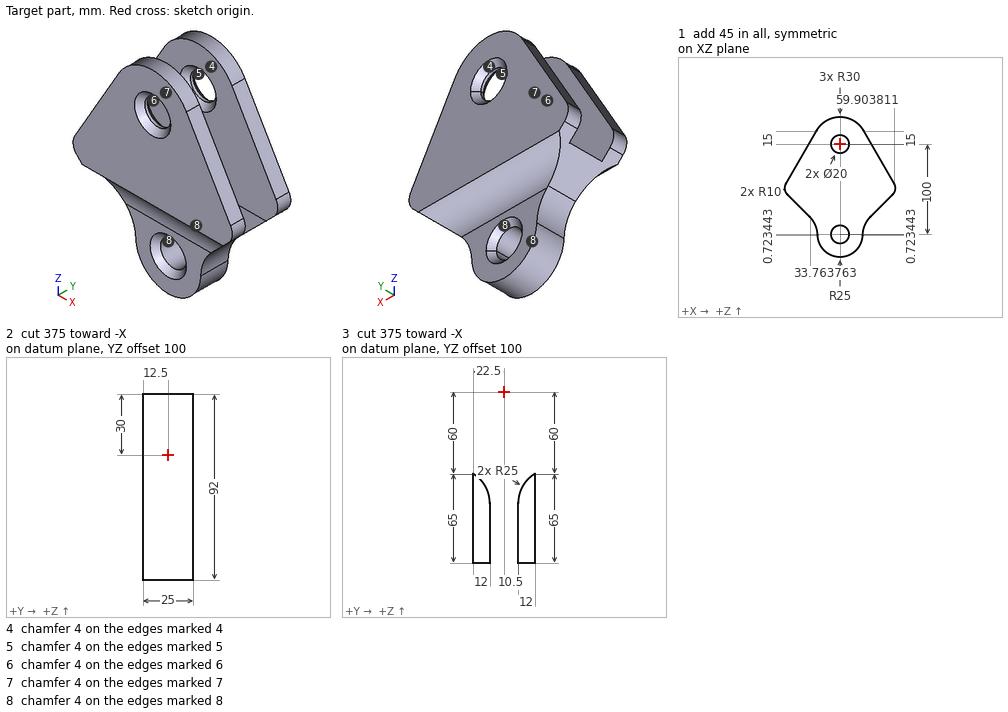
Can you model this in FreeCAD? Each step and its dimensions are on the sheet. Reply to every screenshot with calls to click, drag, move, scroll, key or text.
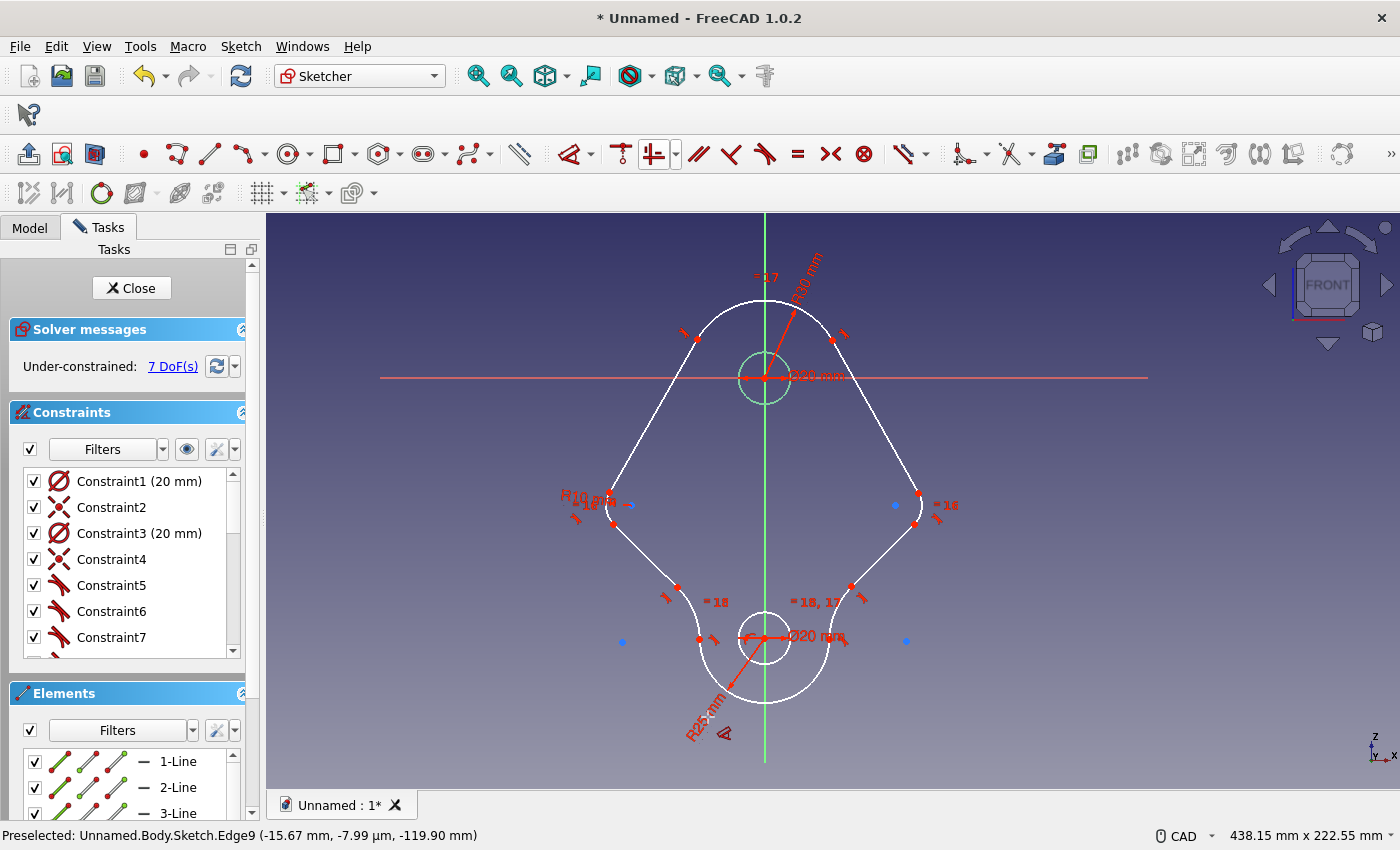
click(697, 340)
click(663, 359)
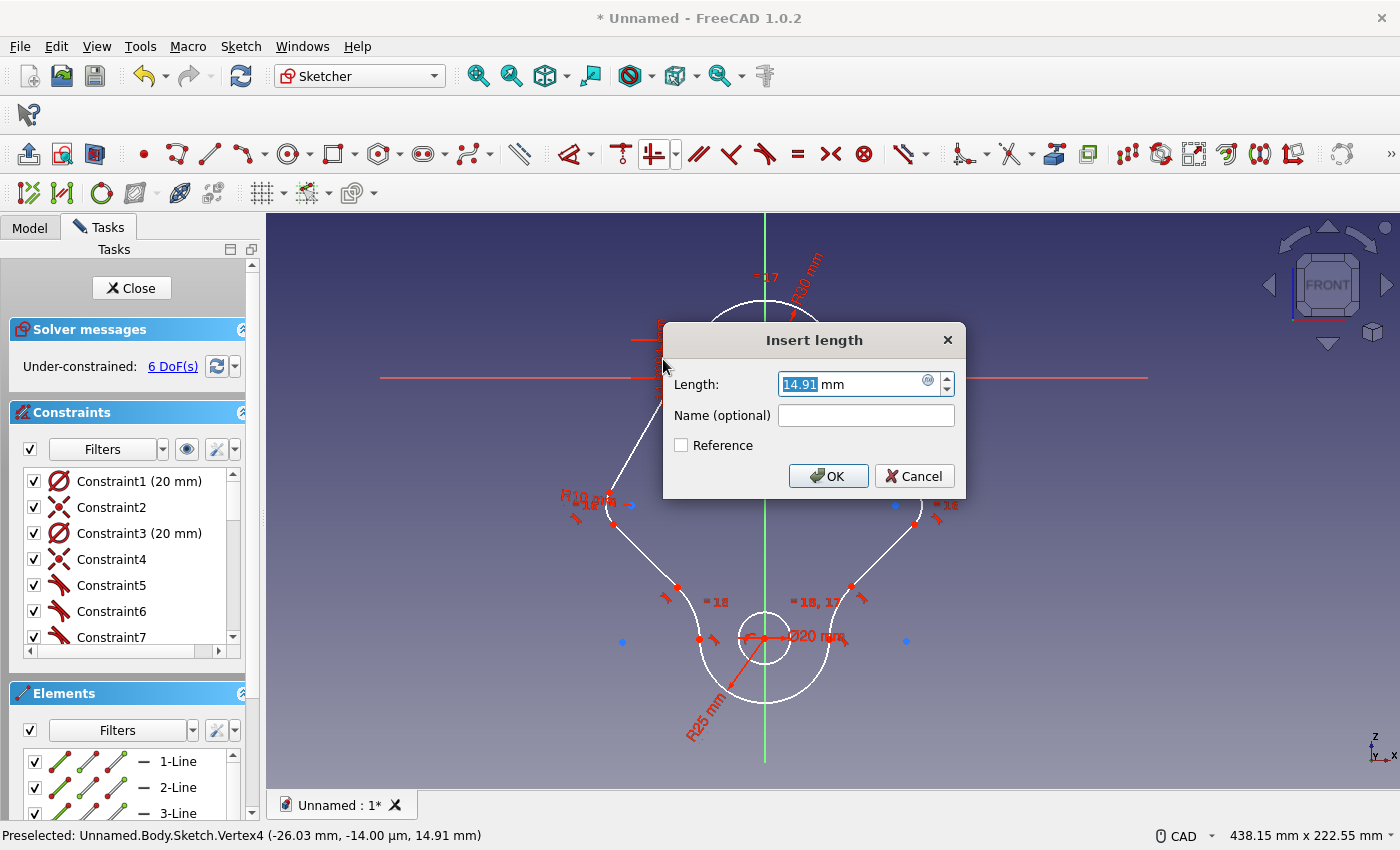
text(15)
key(Return)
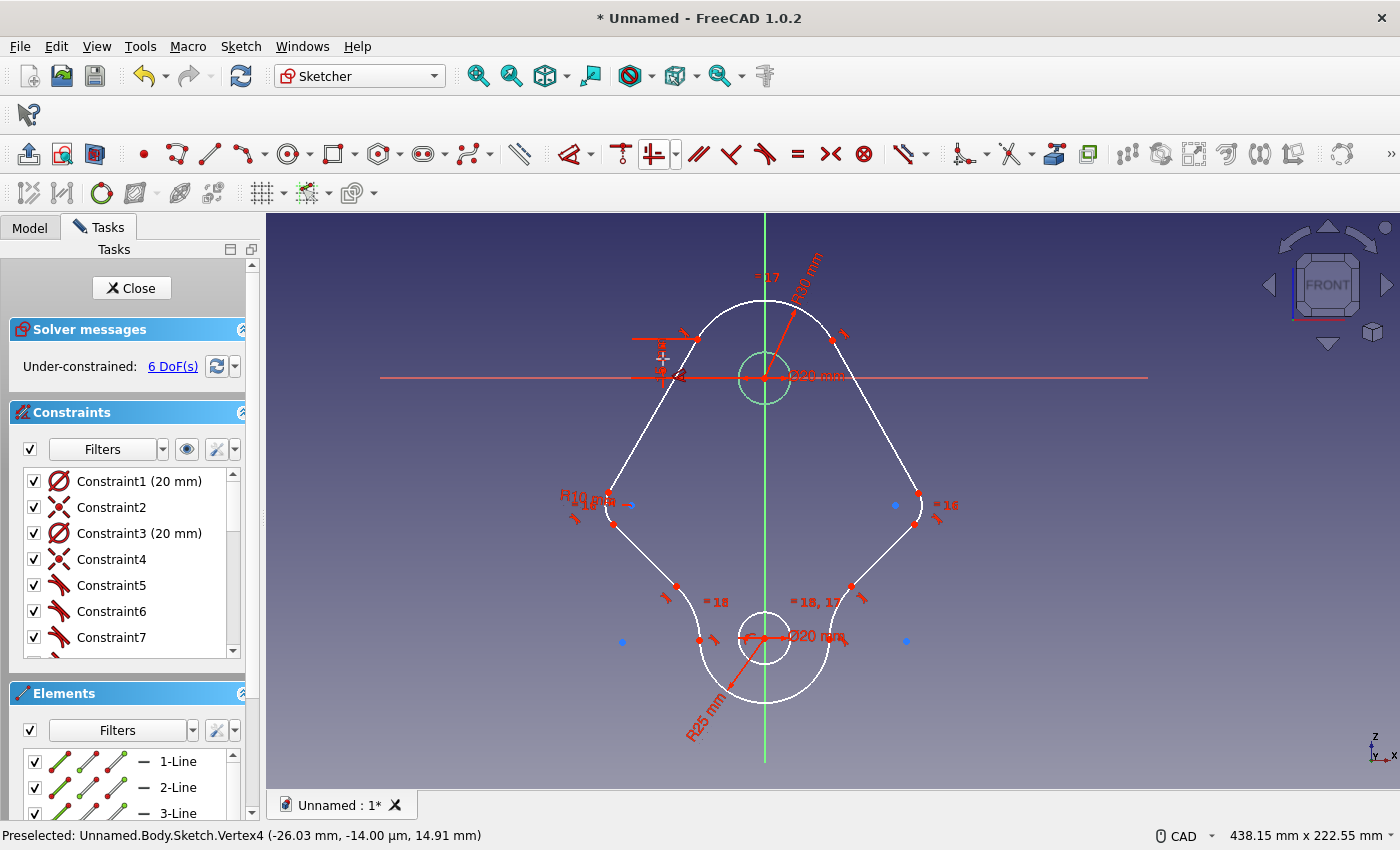
click(832, 340)
click(866, 359)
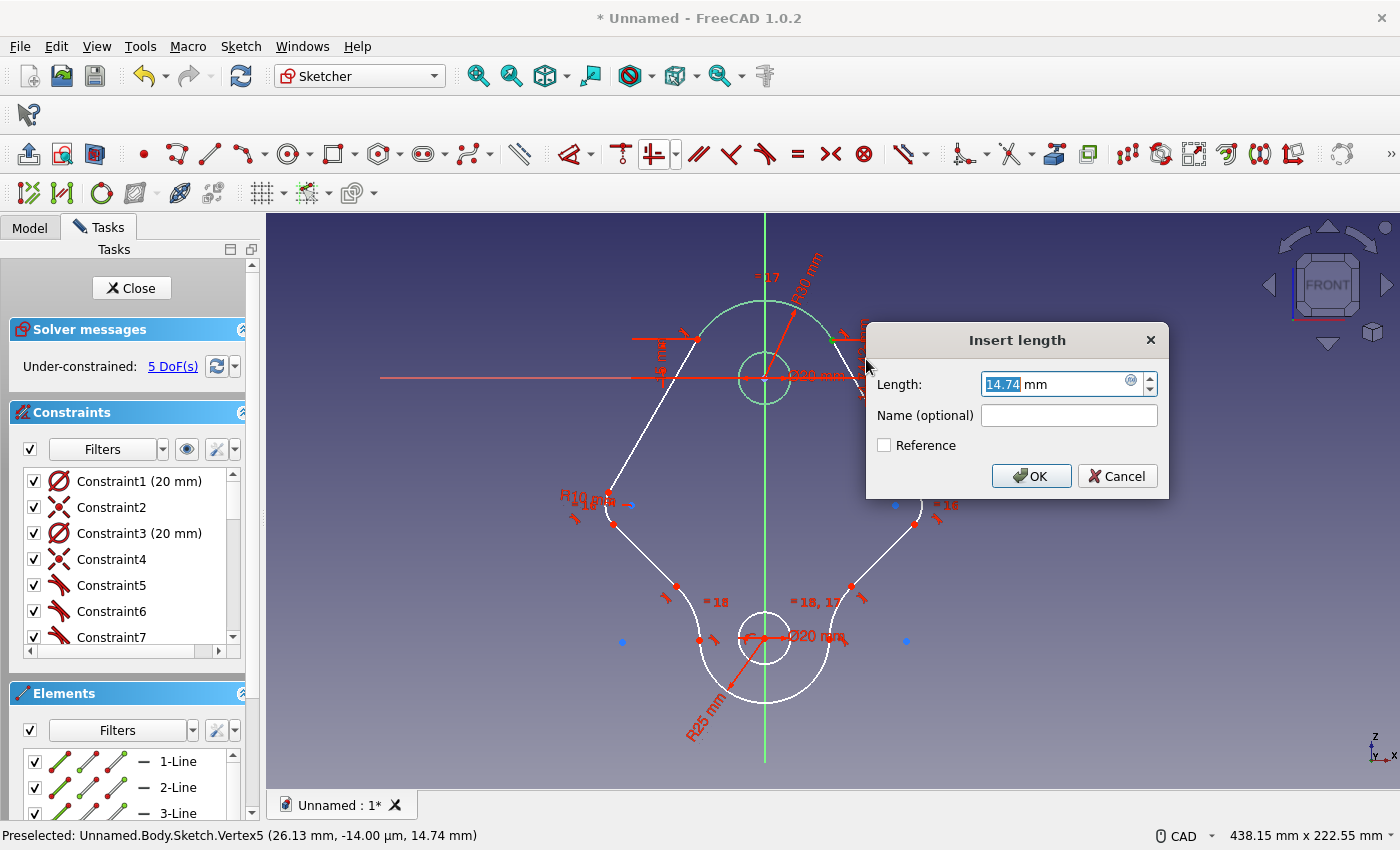
text(15)
key(Return)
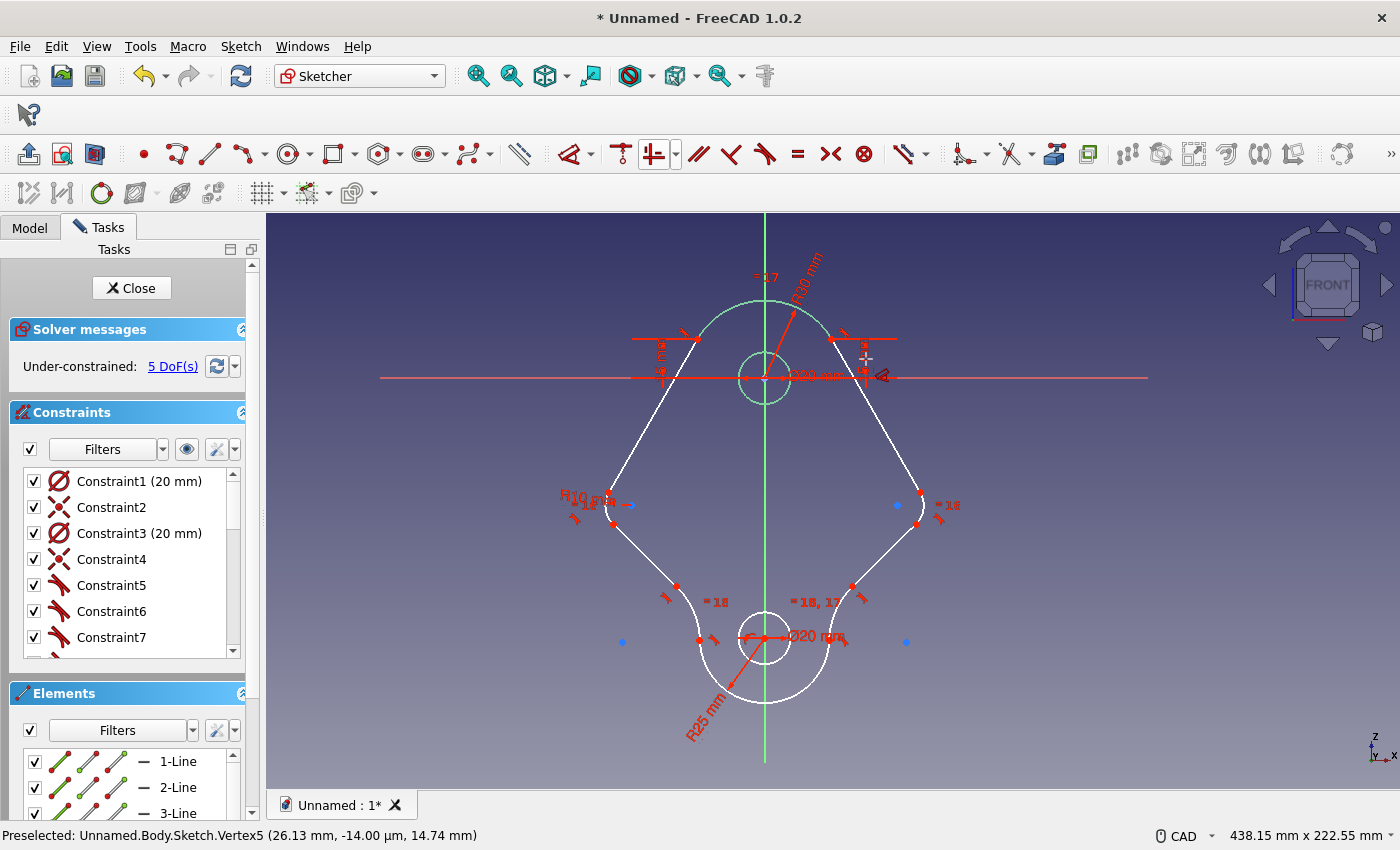
click(765, 638)
click(799, 508)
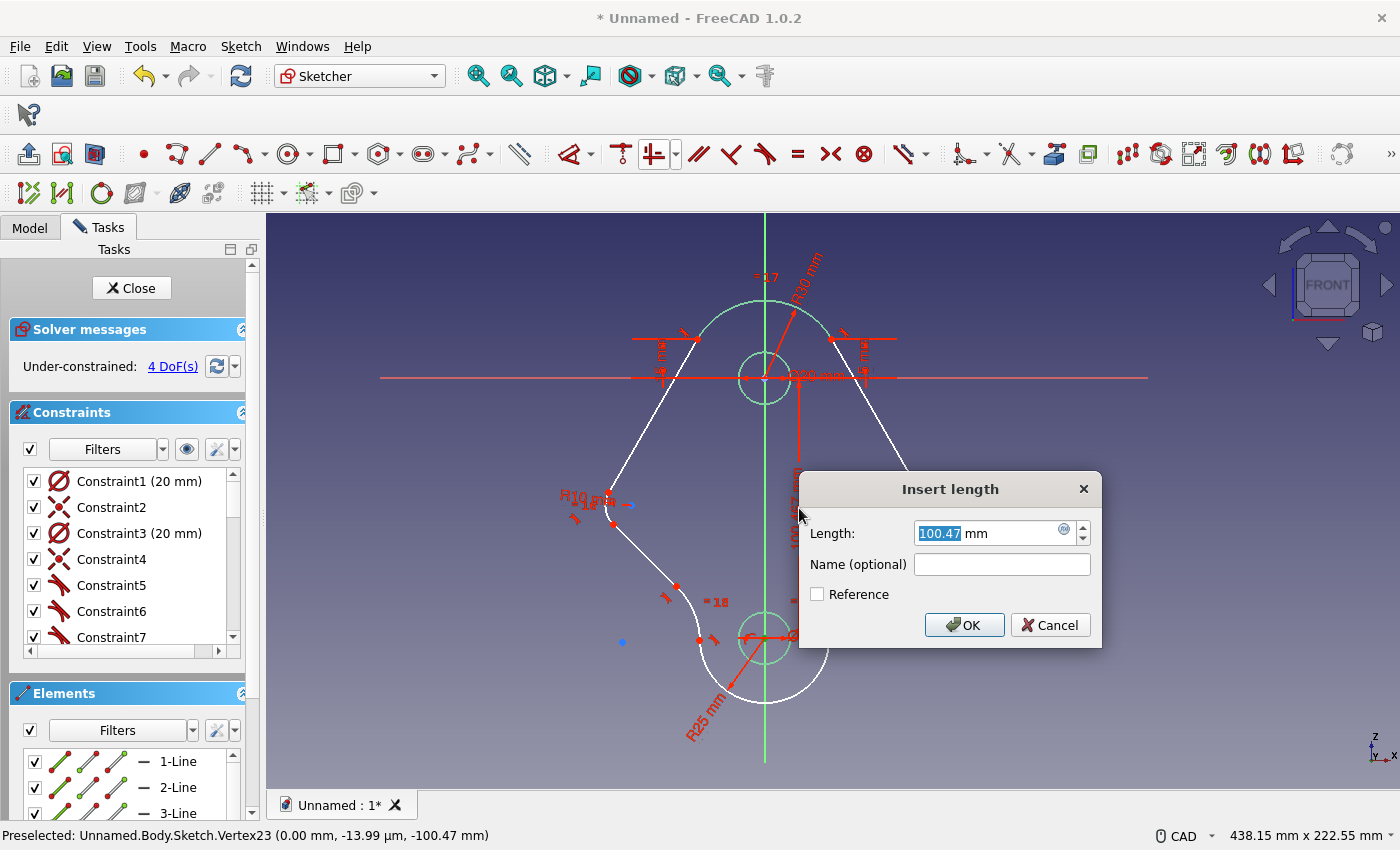
text(100)
key(Return)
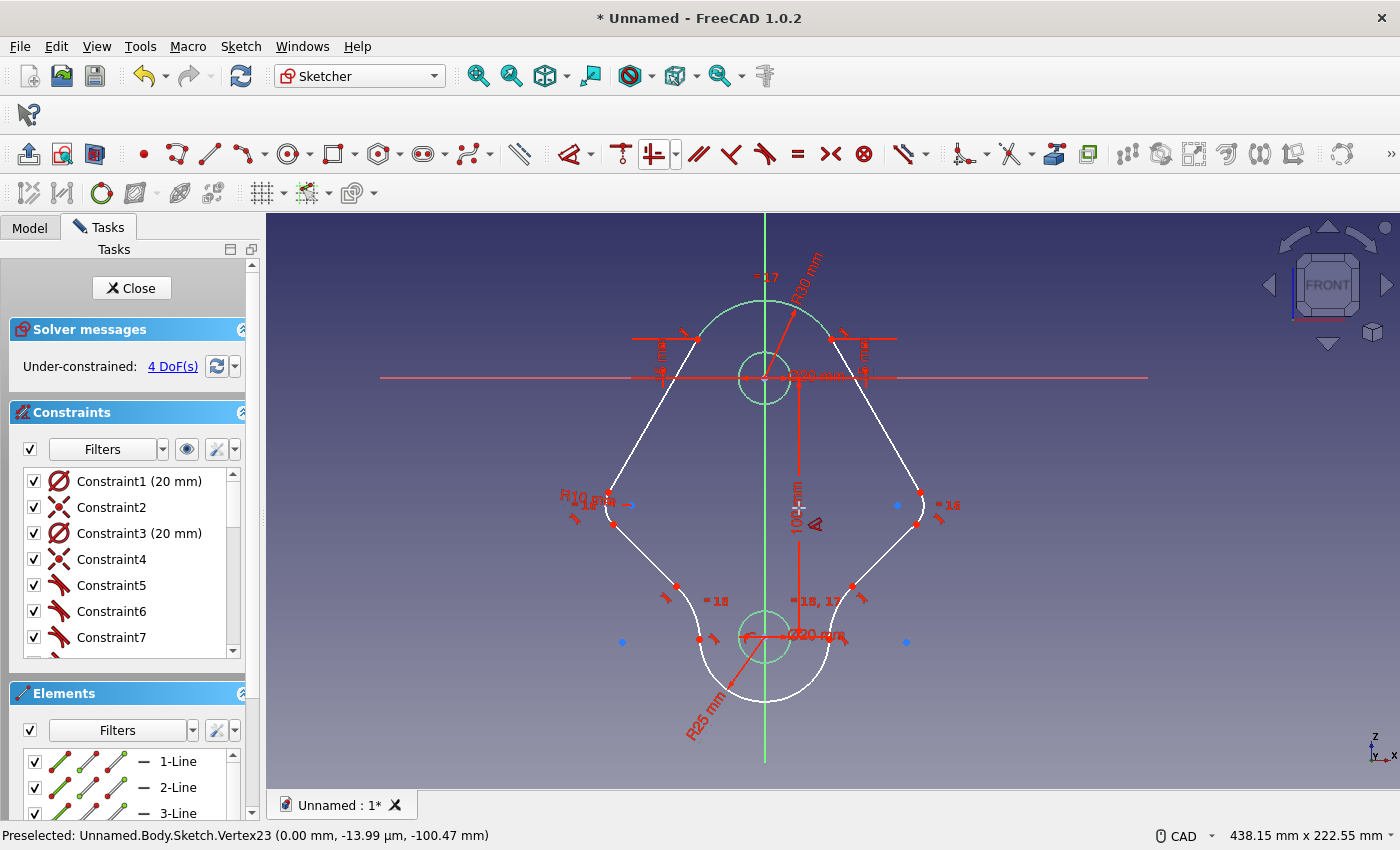
scroll(829, 639, up, 16)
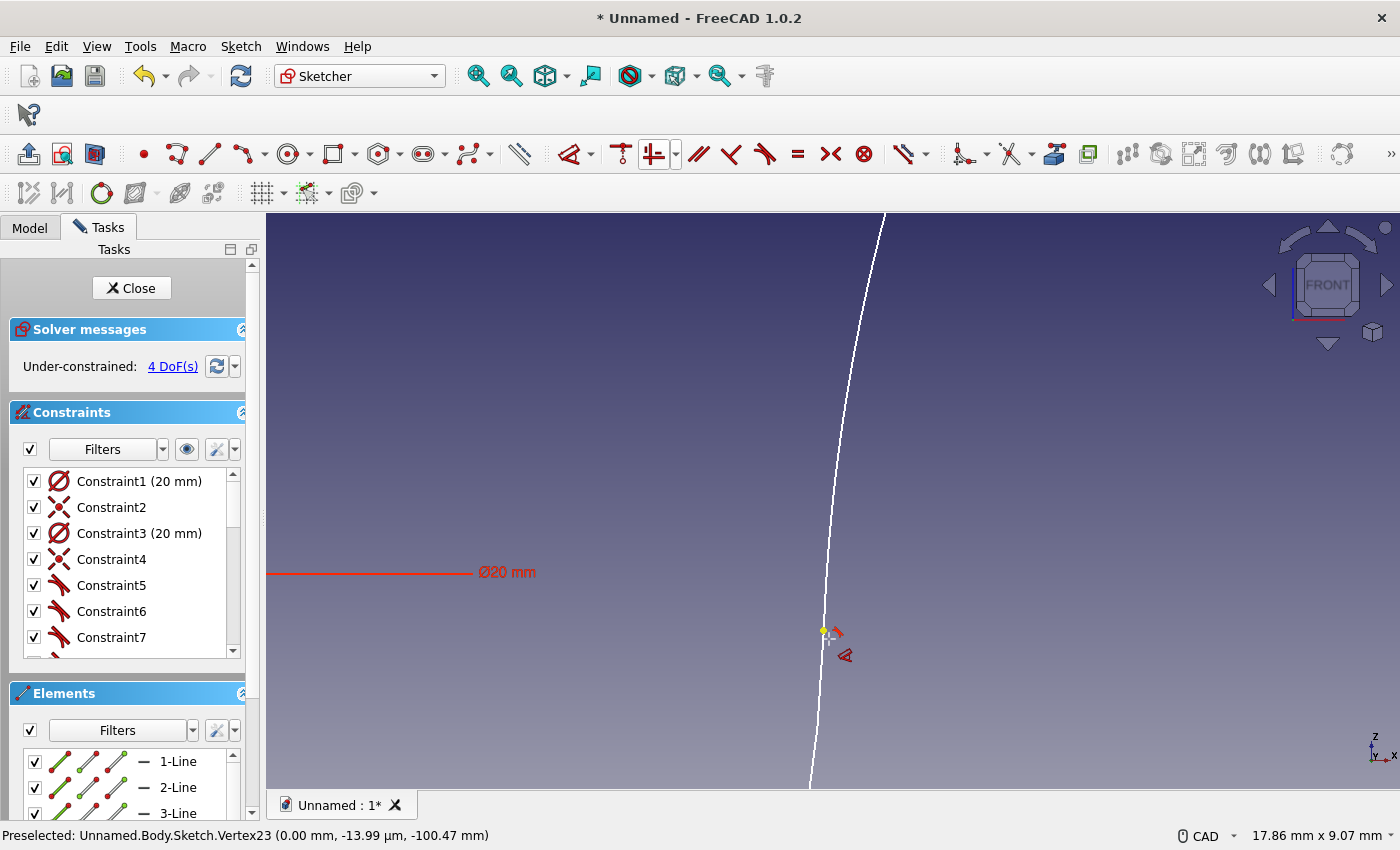
click(824, 631)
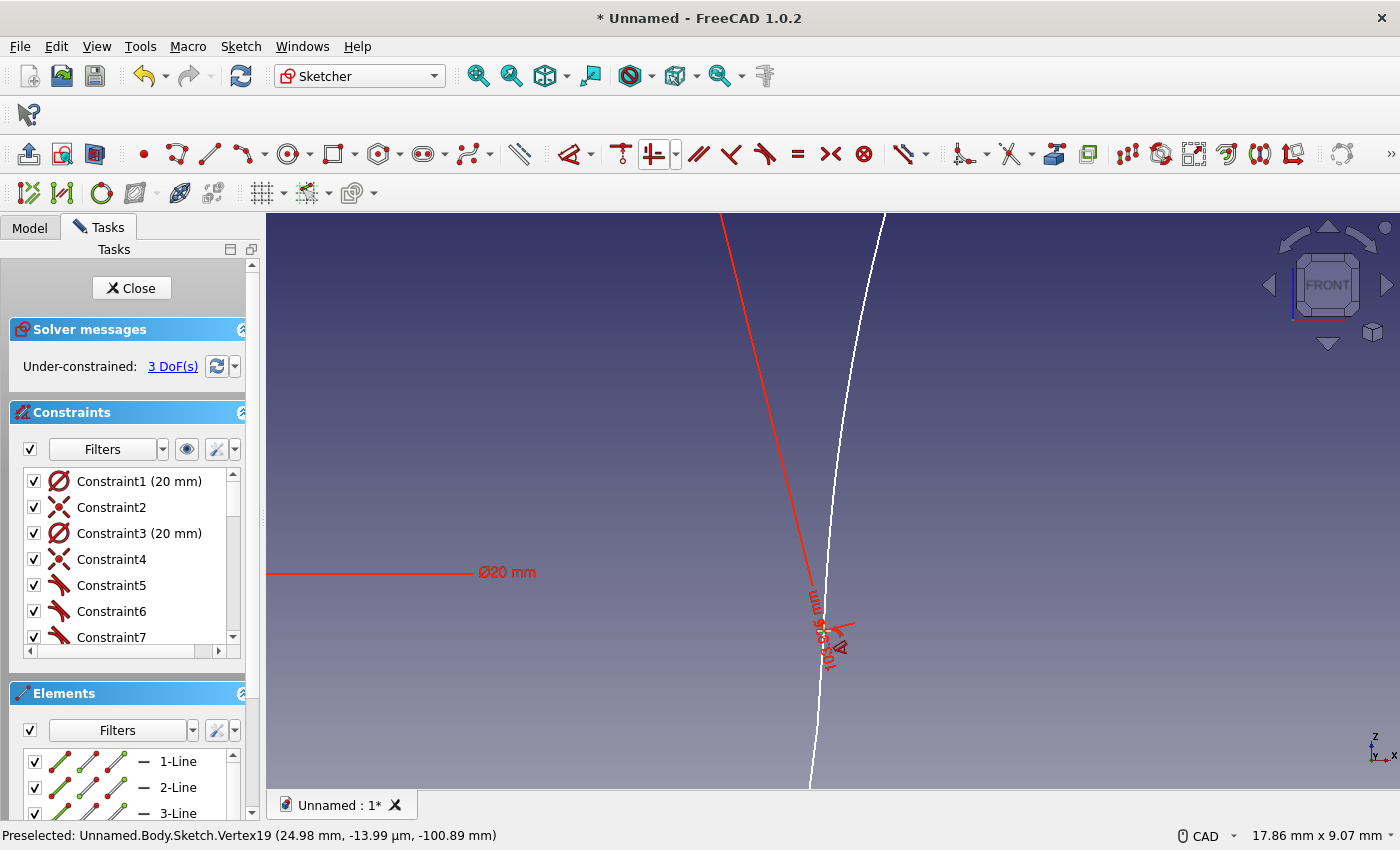
scroll(829, 640, down, 16)